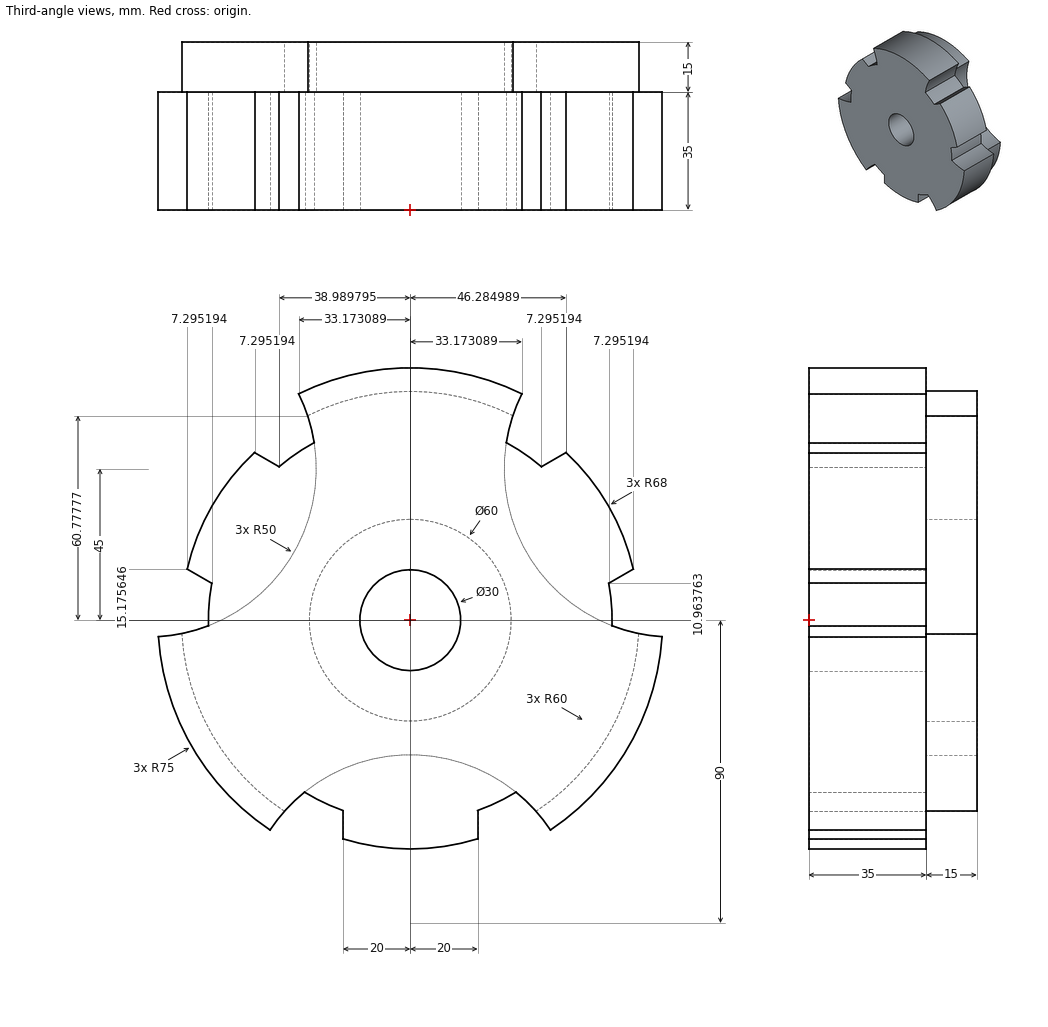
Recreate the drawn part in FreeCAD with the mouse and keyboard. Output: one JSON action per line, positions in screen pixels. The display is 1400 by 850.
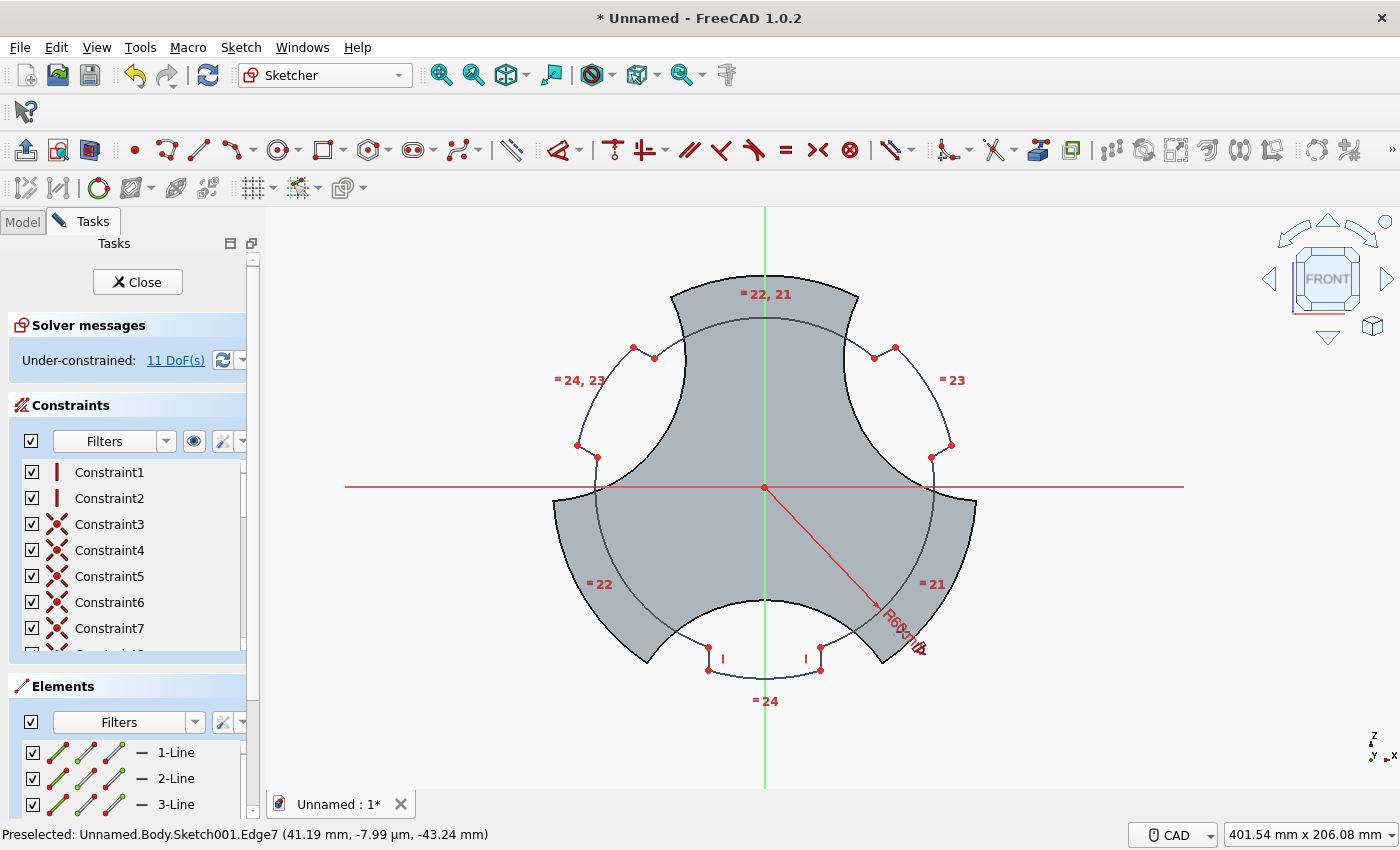
{"action": "left_click", "coordinate": [941, 413]}
{"action": "left_click", "coordinate": [970, 401]}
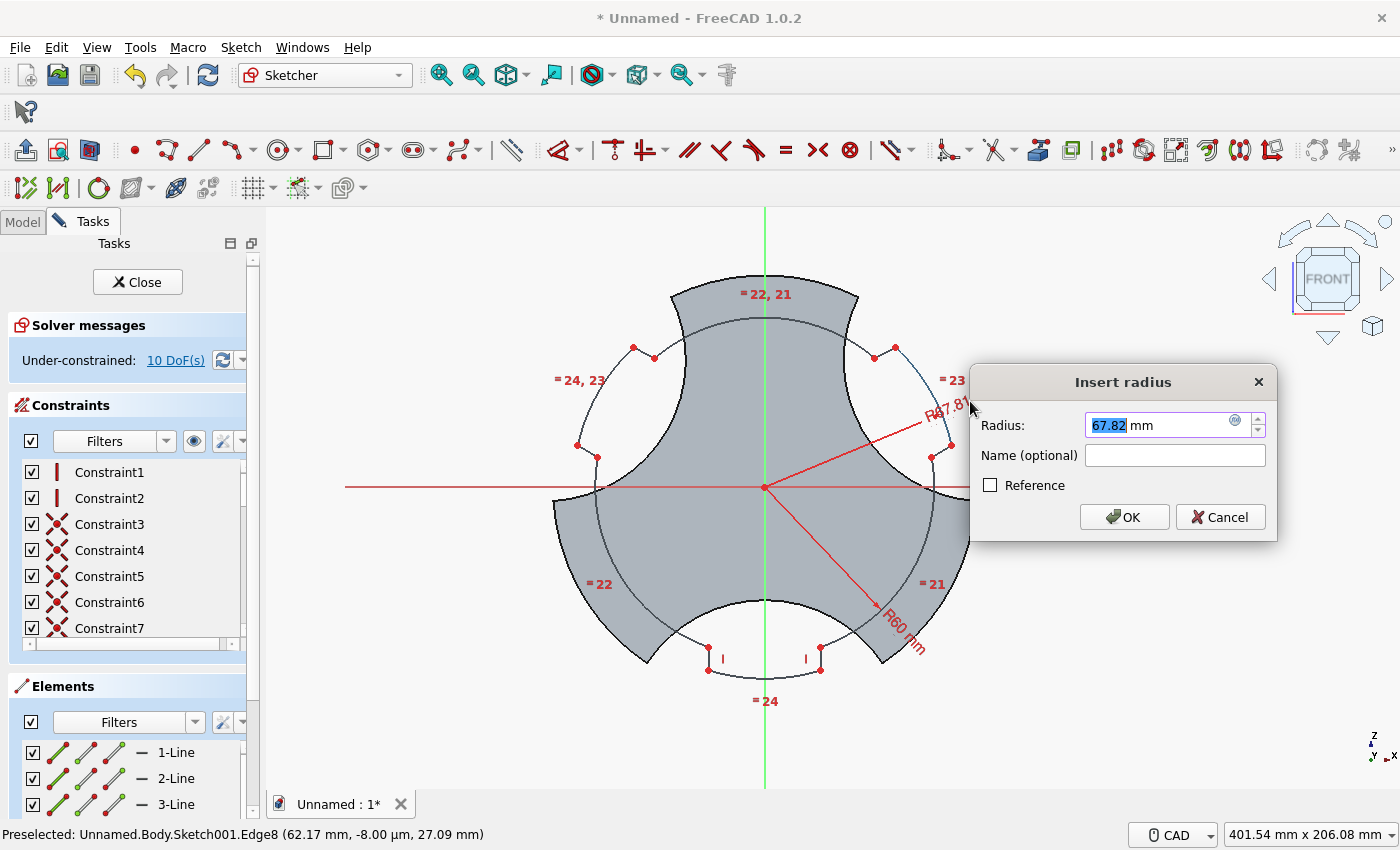
{"action": "type", "text": "68"}
{"action": "key", "text": "Return"}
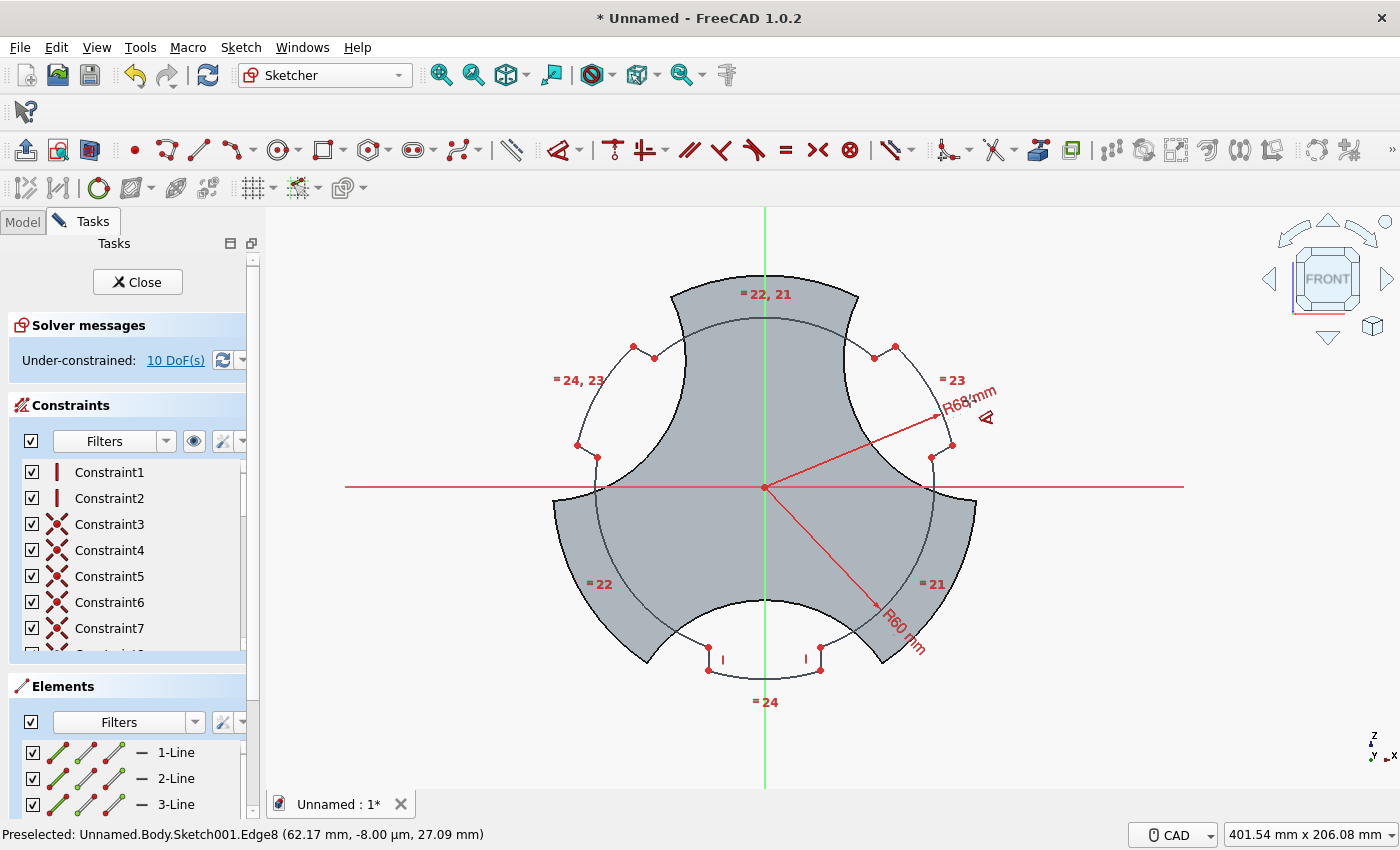
{"action": "left_click", "coordinate": [821, 671]}
{"action": "left_click", "coordinate": [793, 705]}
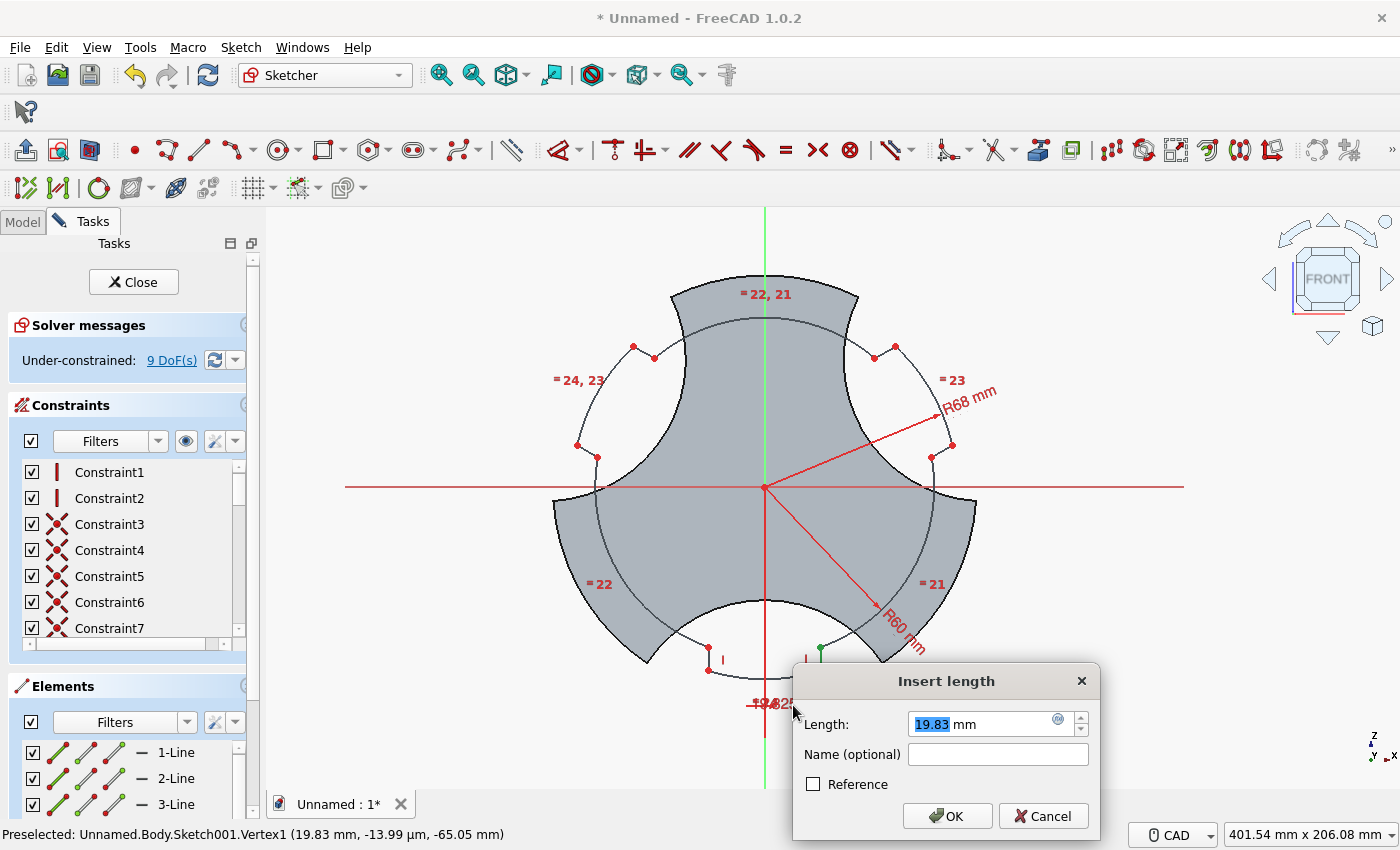
{"action": "type", "text": "20"}
{"action": "key", "text": "Return"}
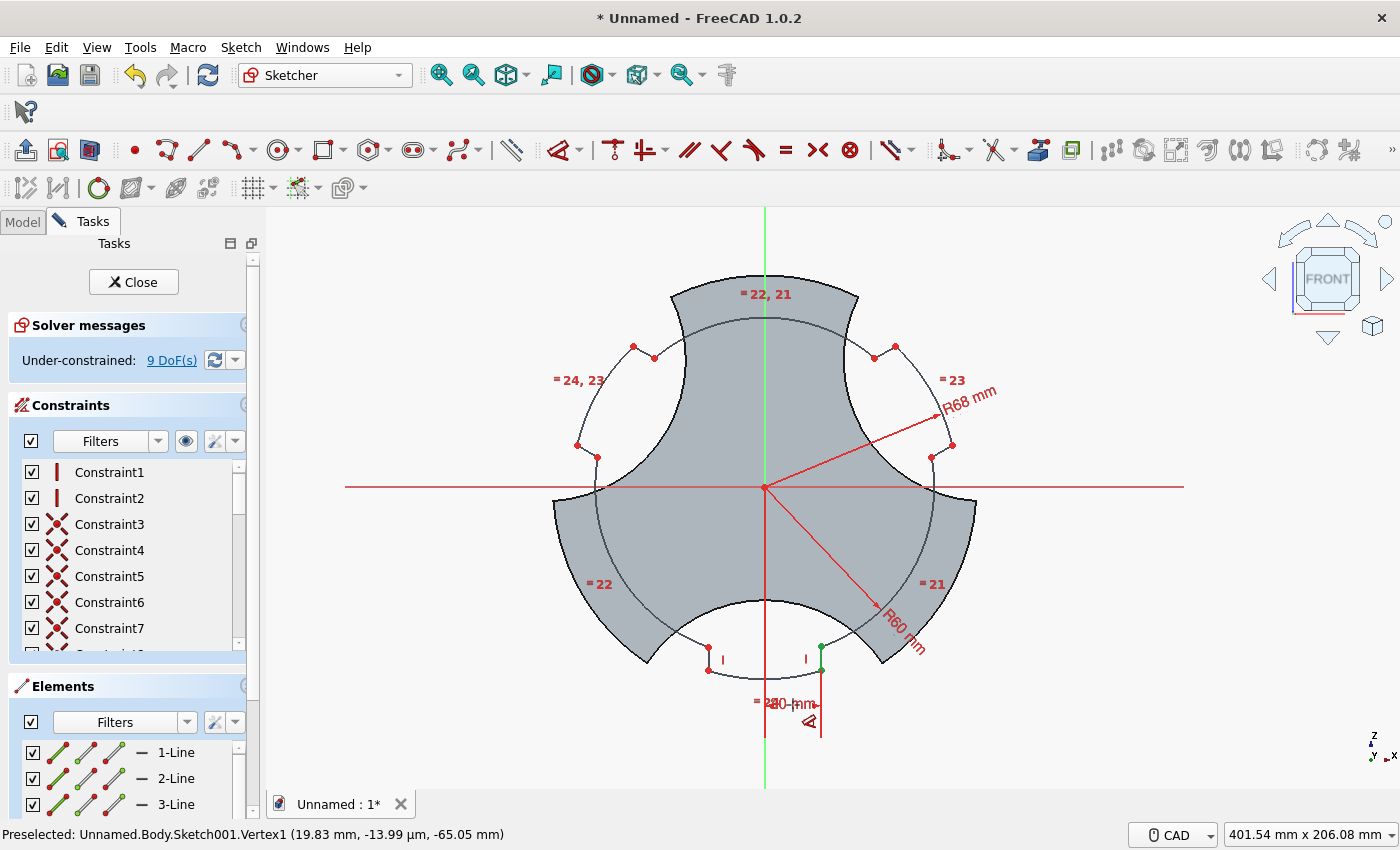
{"action": "left_click", "coordinate": [709, 647]}
{"action": "left_click", "coordinate": [737, 453]}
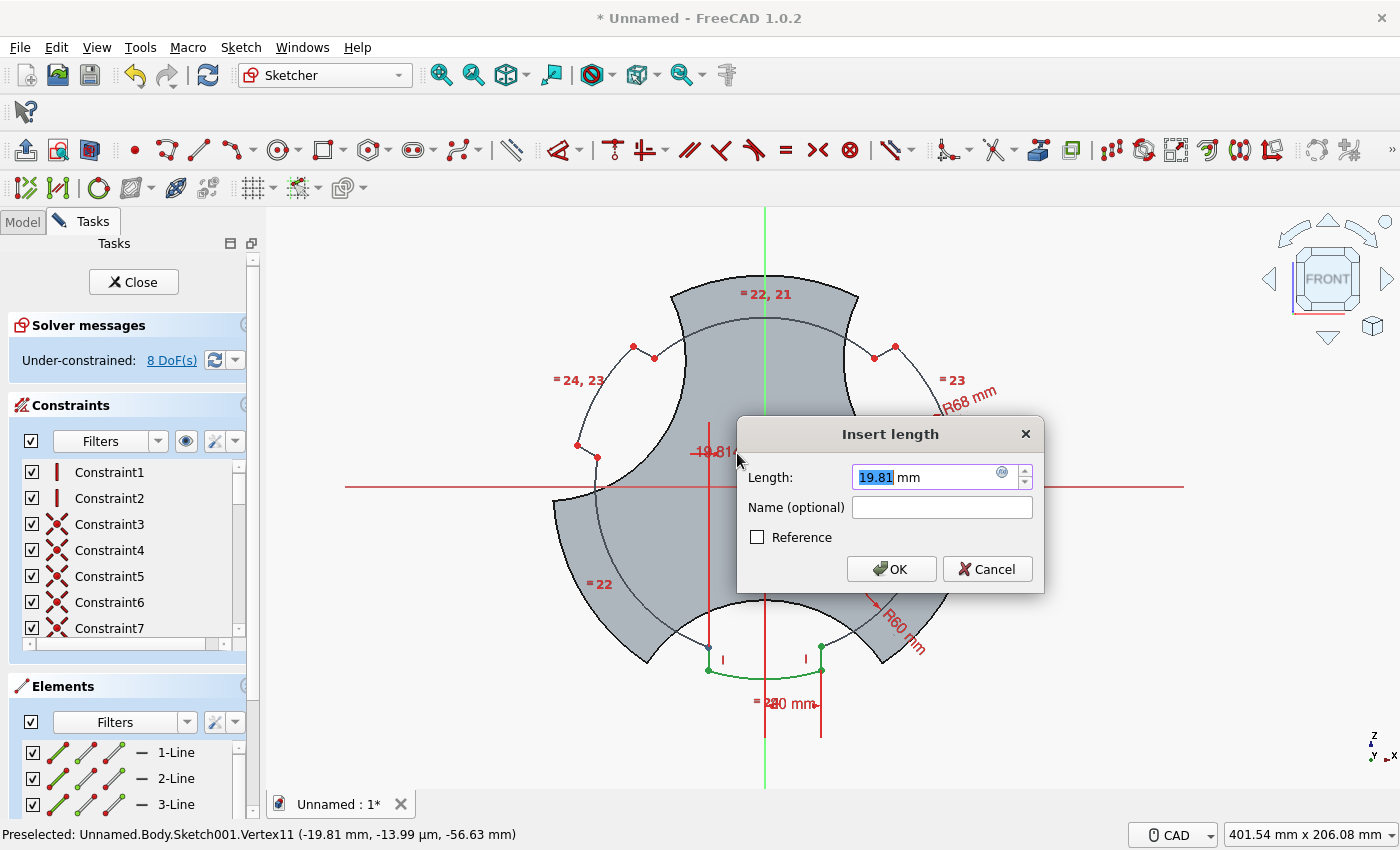
{"action": "type", "text": "20"}
{"action": "key", "text": "Return"}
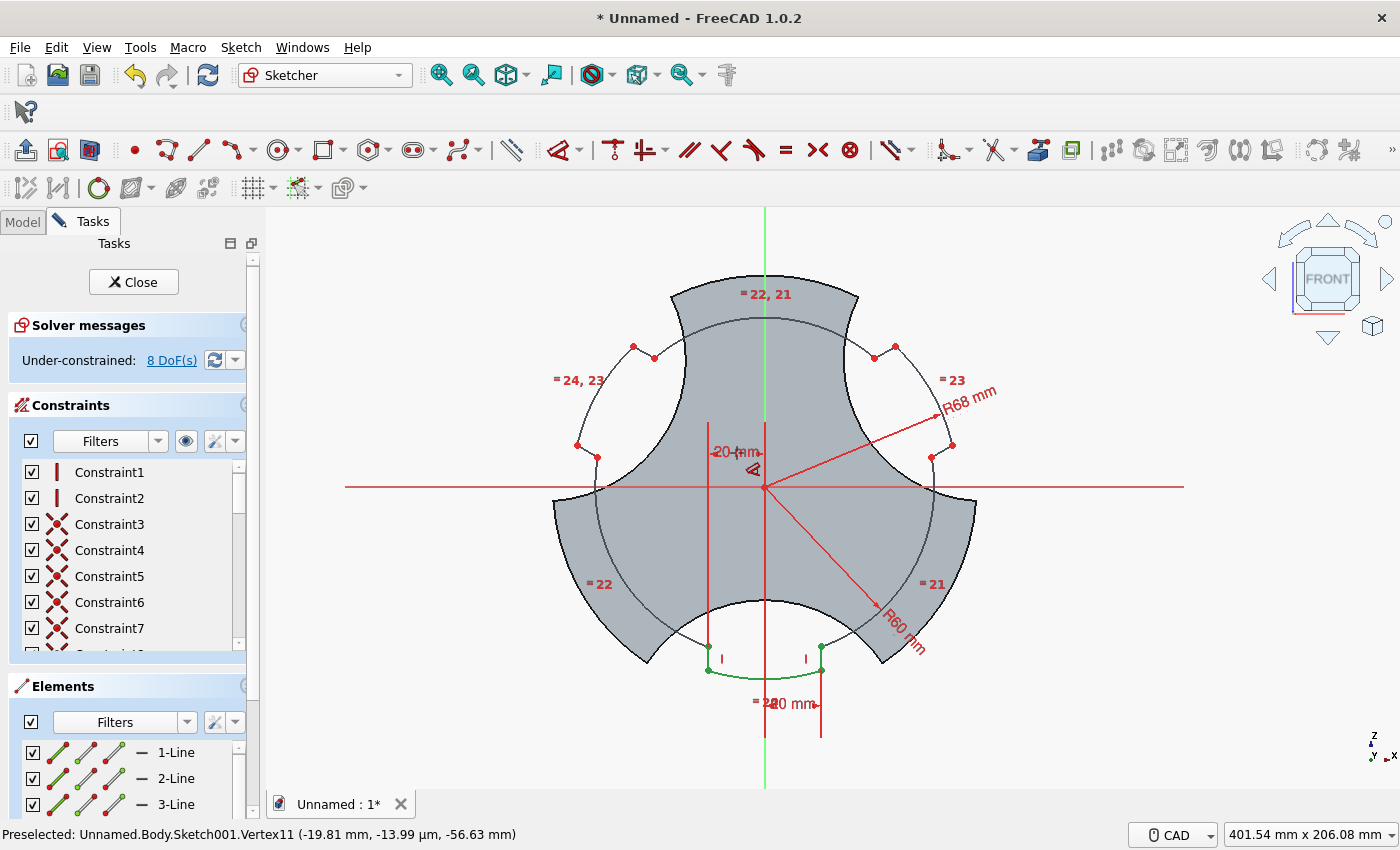
{"action": "scroll", "coordinate": [940, 453], "scroll_direction": "up", "scroll_amount": 4}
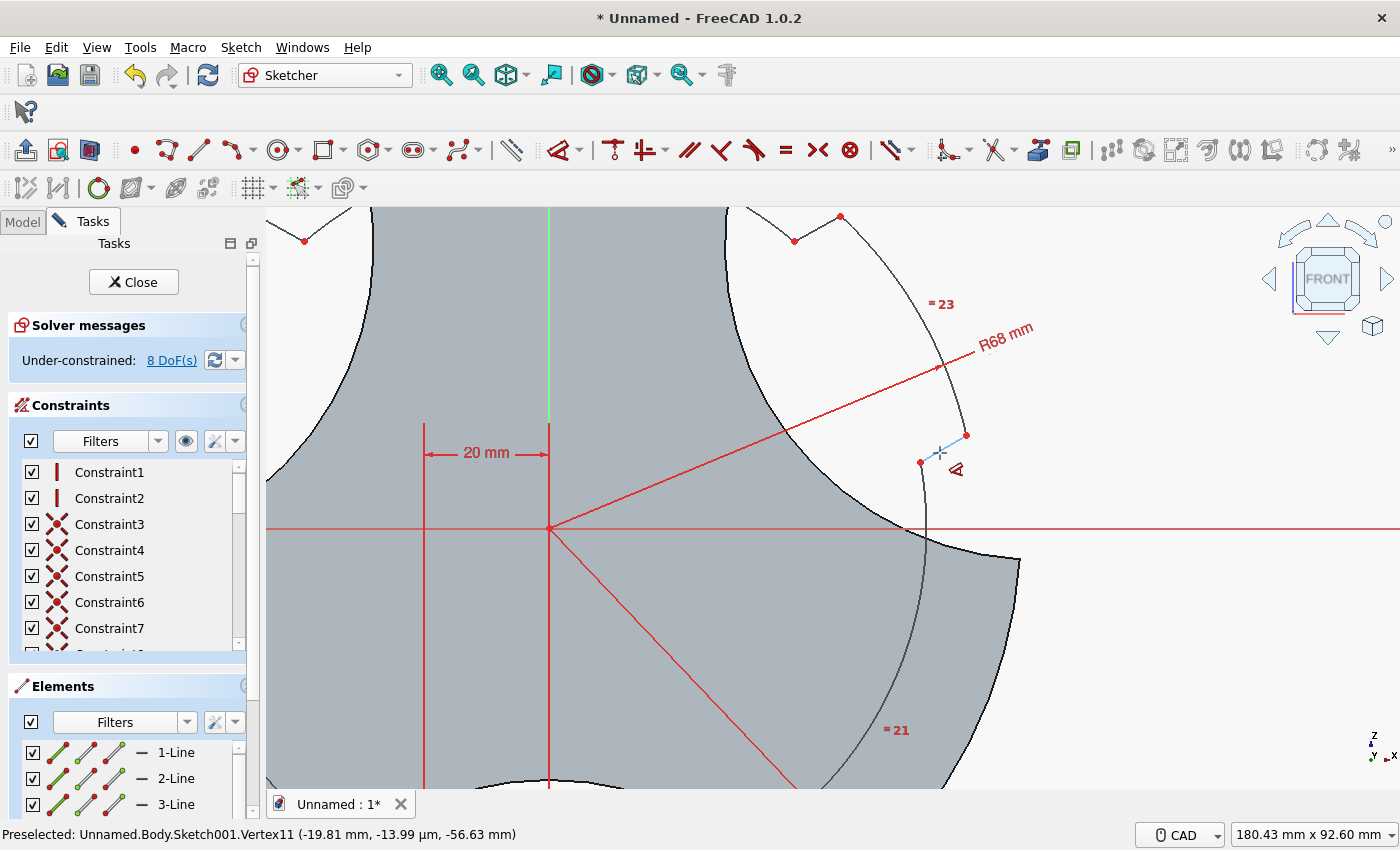
{"action": "left_click", "coordinate": [939, 452]}
{"action": "left_click", "coordinate": [943, 402]}